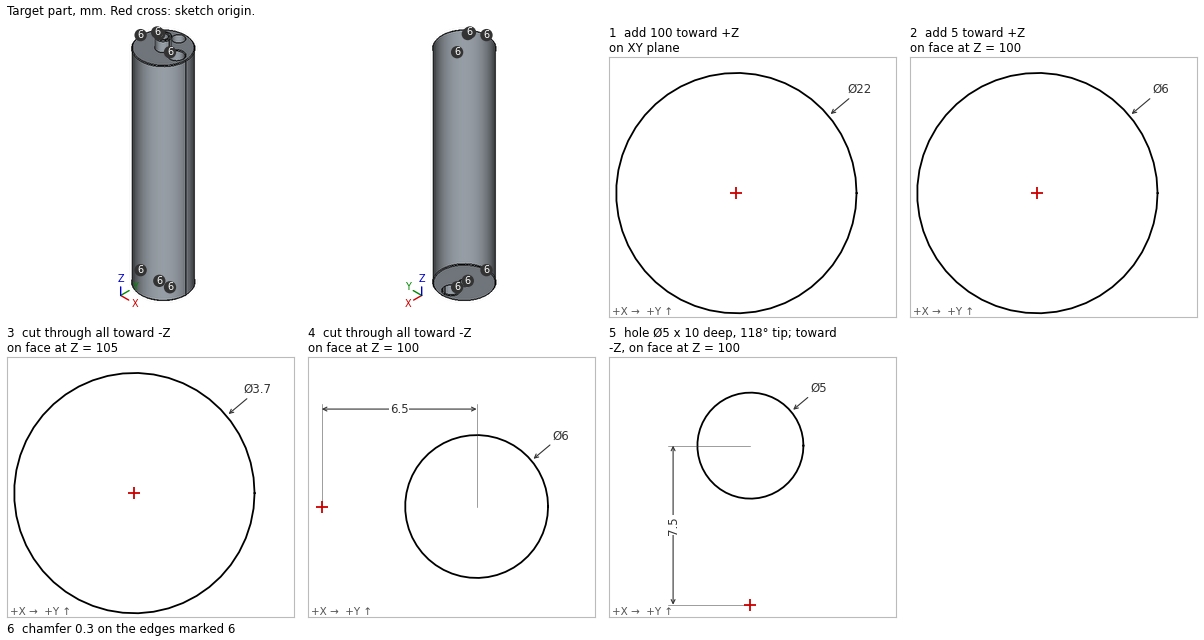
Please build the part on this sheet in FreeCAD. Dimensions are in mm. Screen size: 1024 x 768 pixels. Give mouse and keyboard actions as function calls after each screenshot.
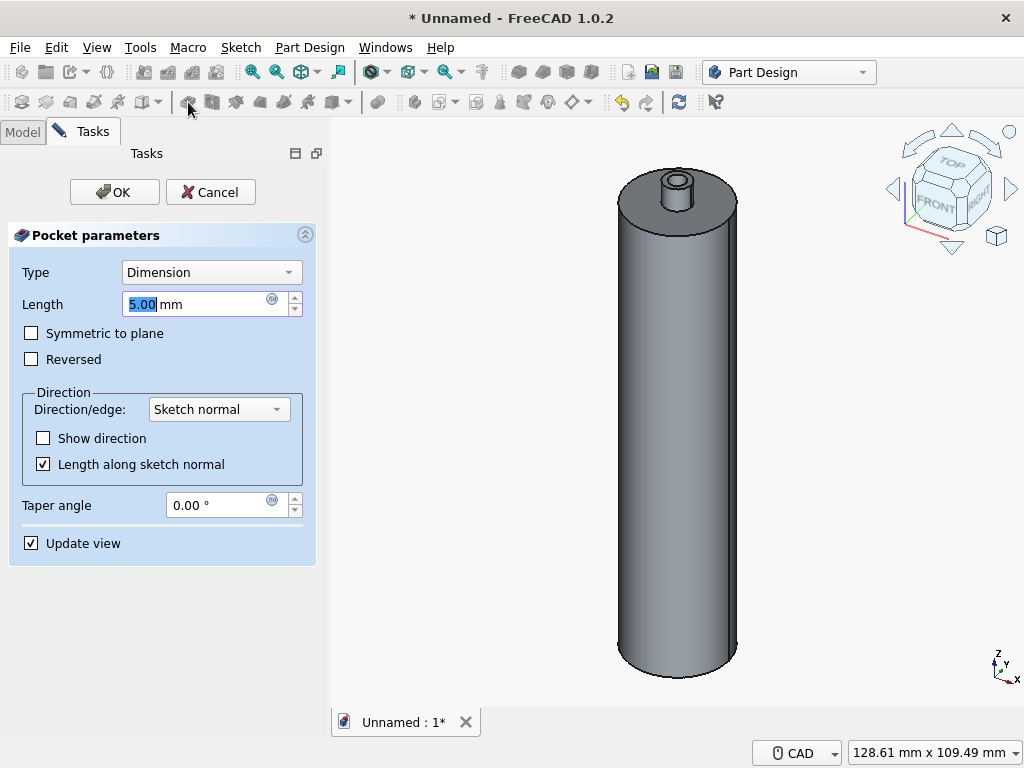
click(212, 272)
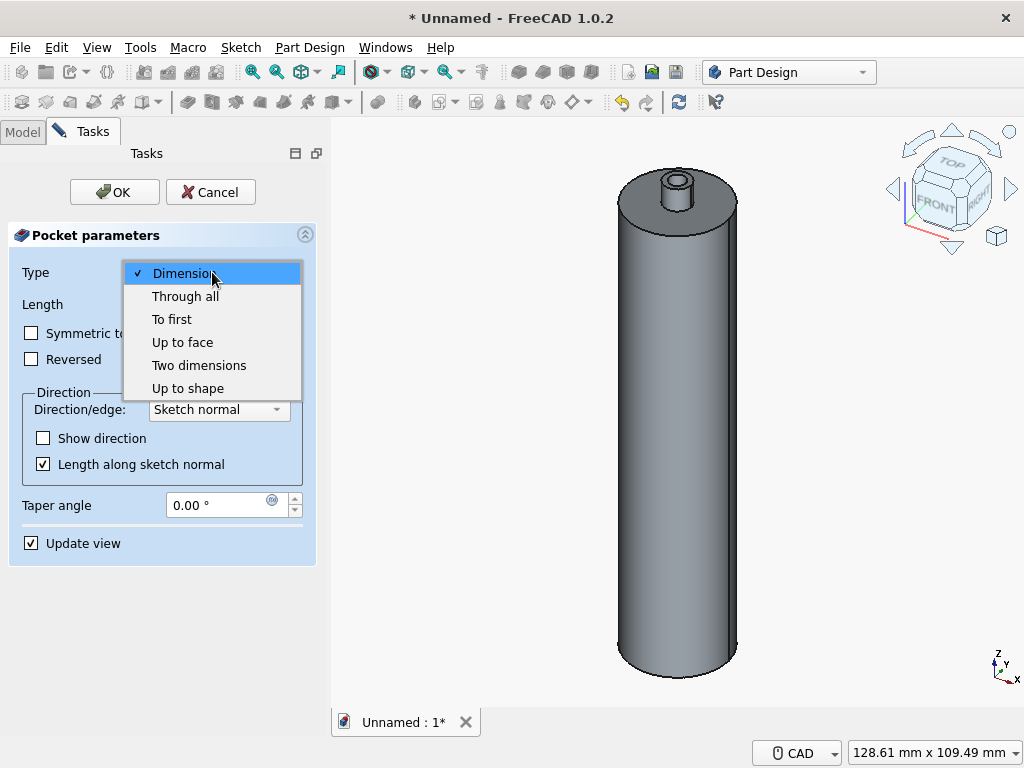
click(212, 296)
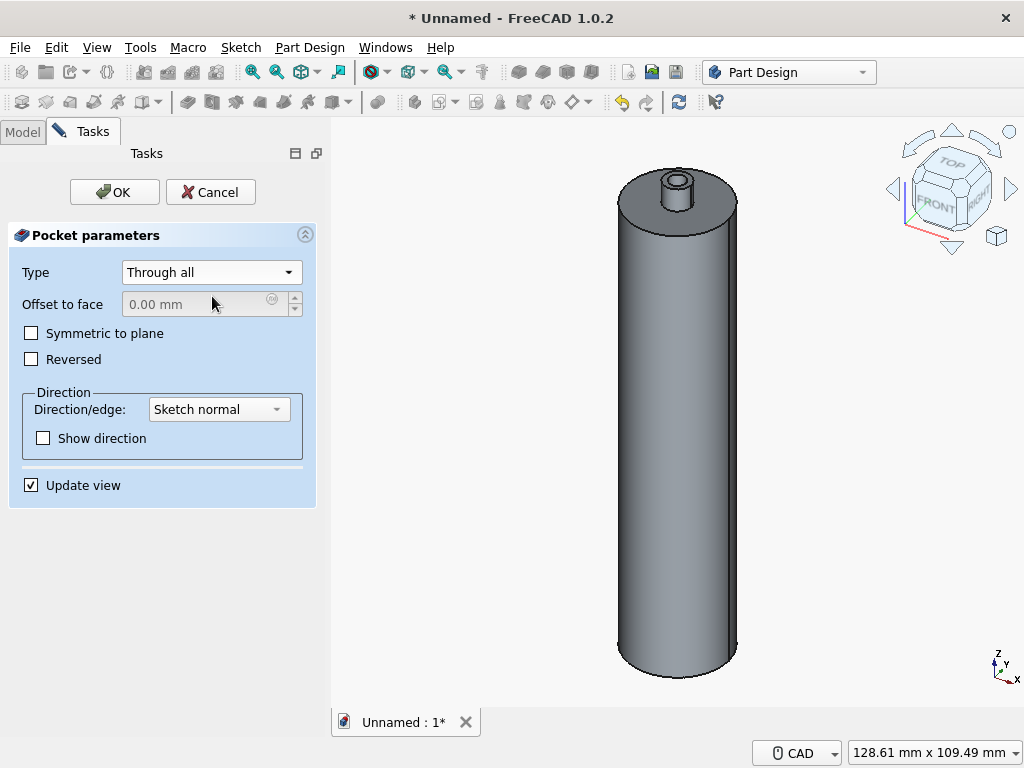
click(115, 192)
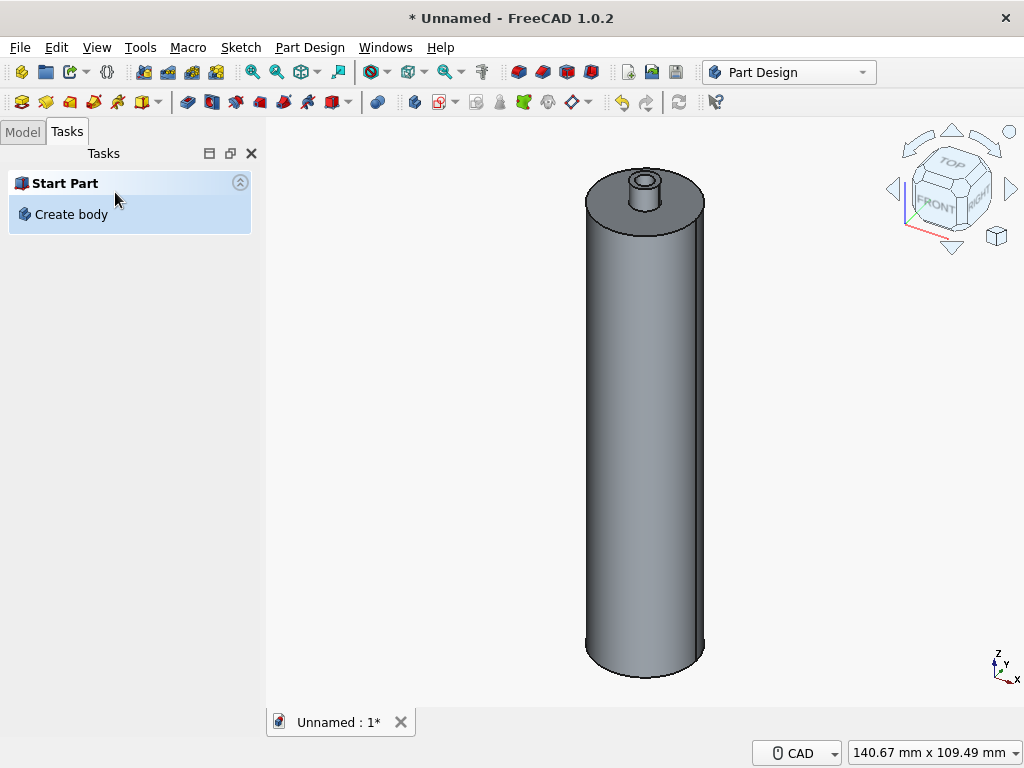
click(677, 189)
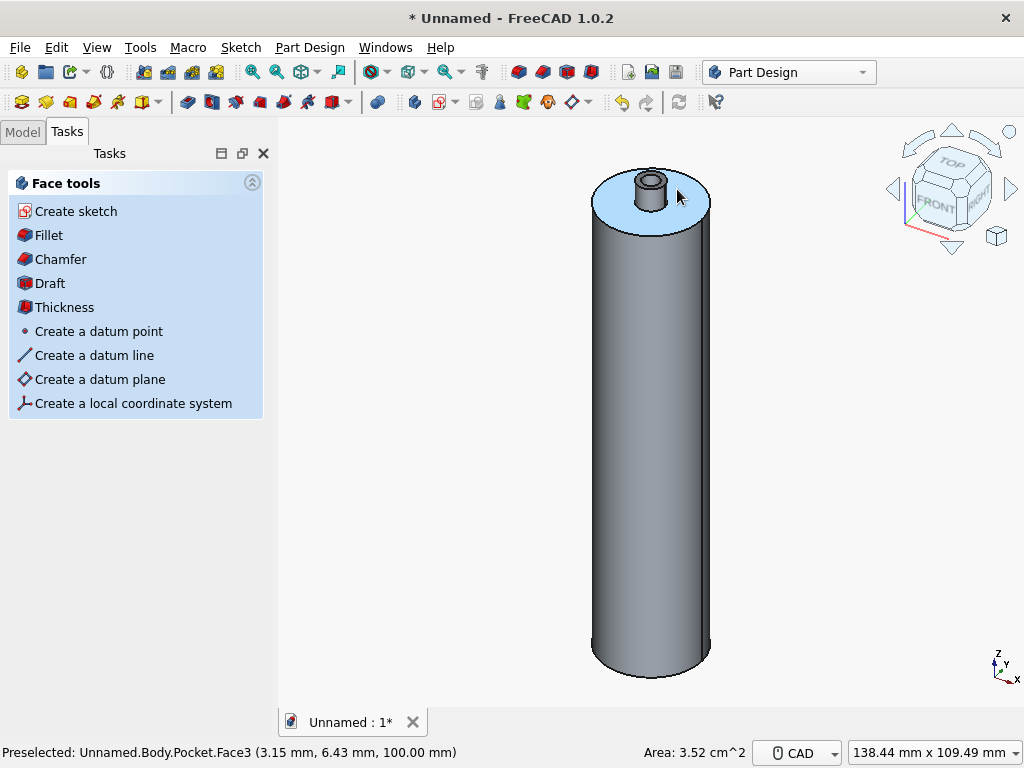
click(440, 102)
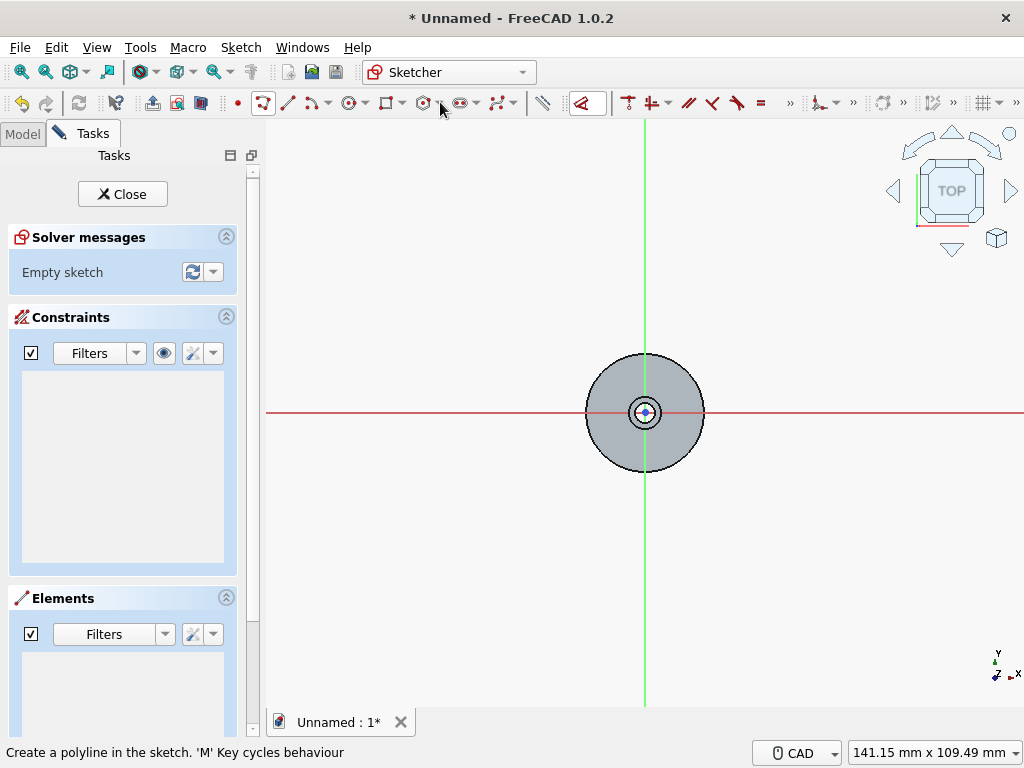
click(202, 104)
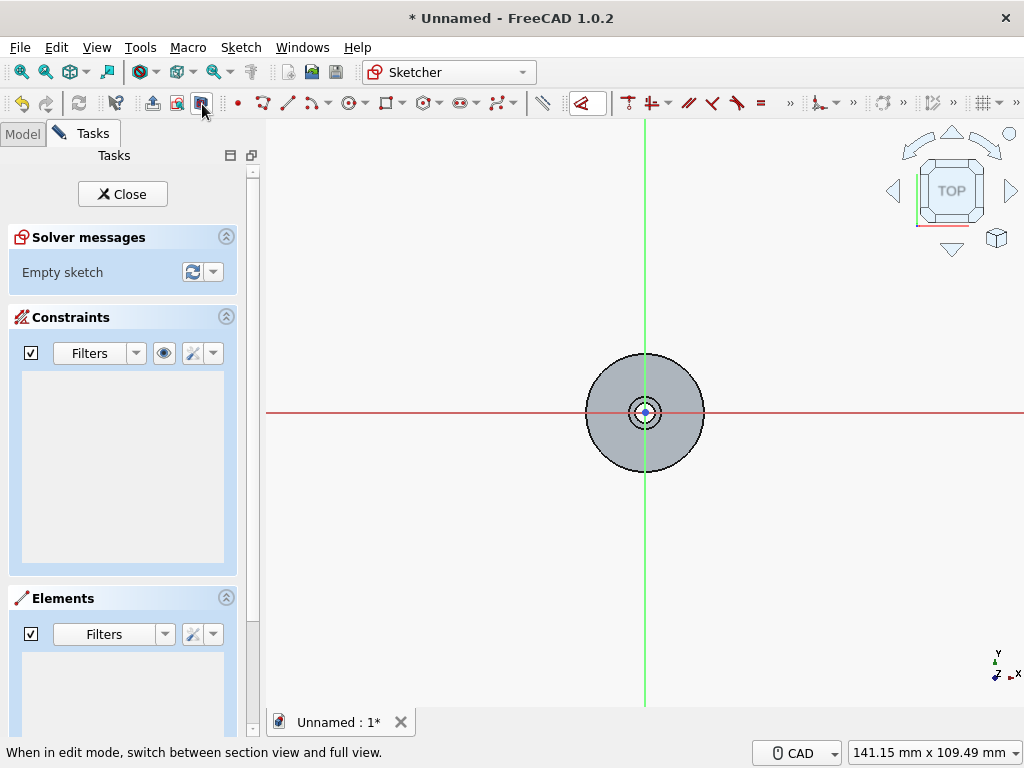
scroll(685, 413, up, 10)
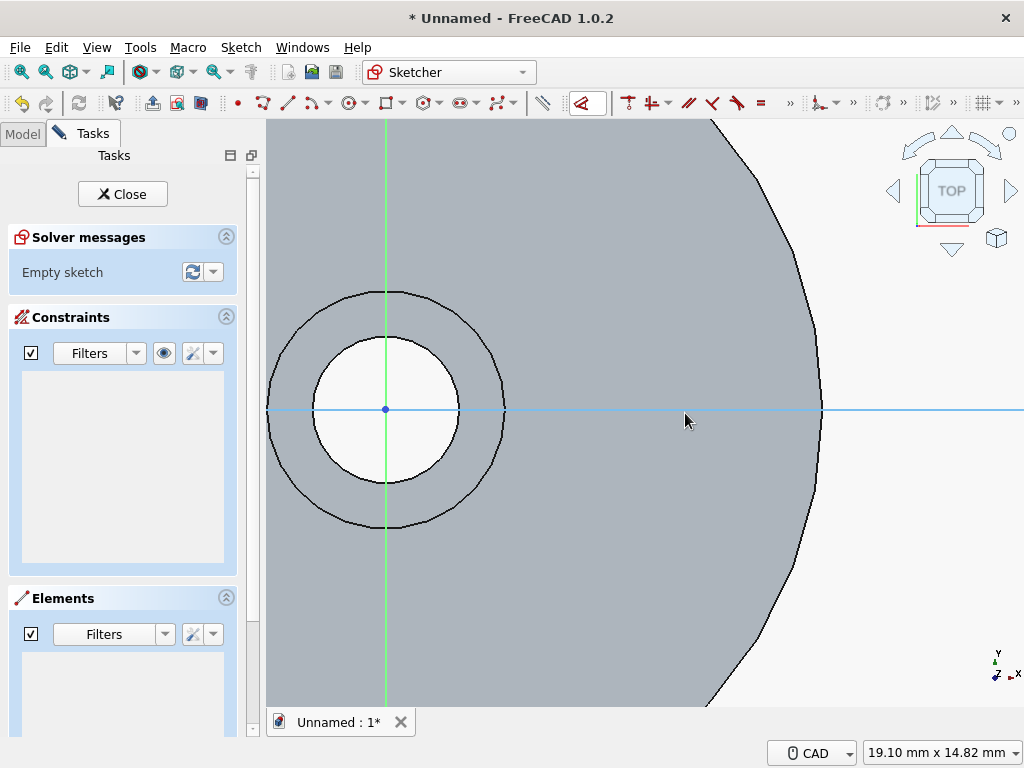
key(g)
key(c)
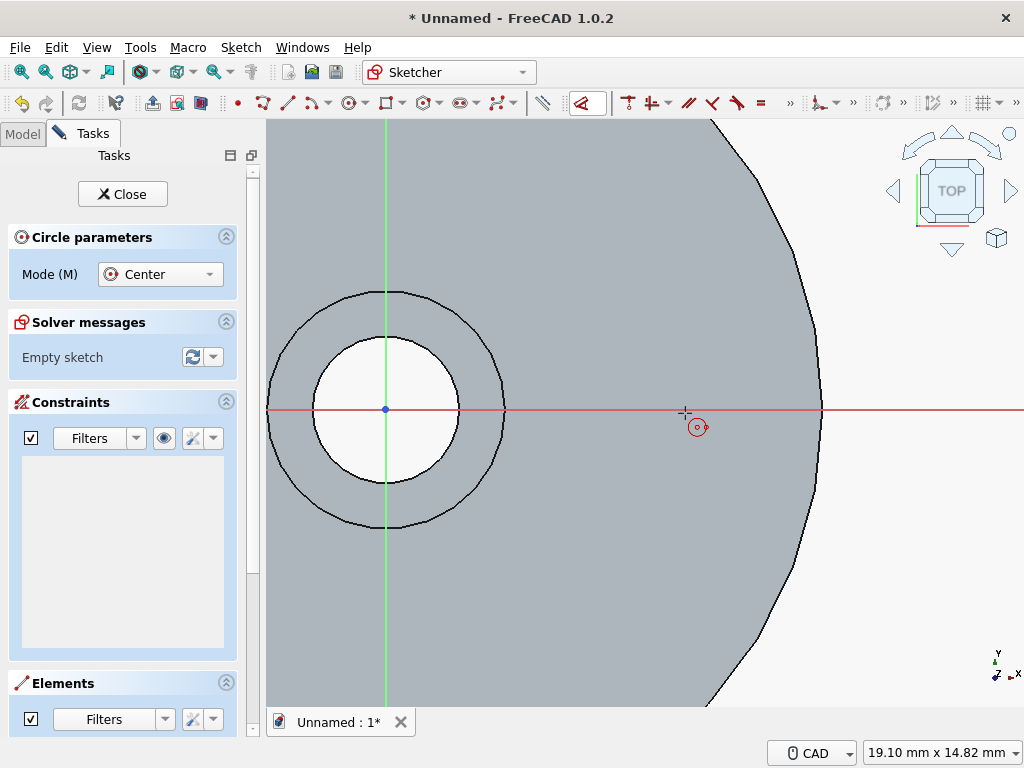
click(644, 410)
click(728, 326)
key(Escape)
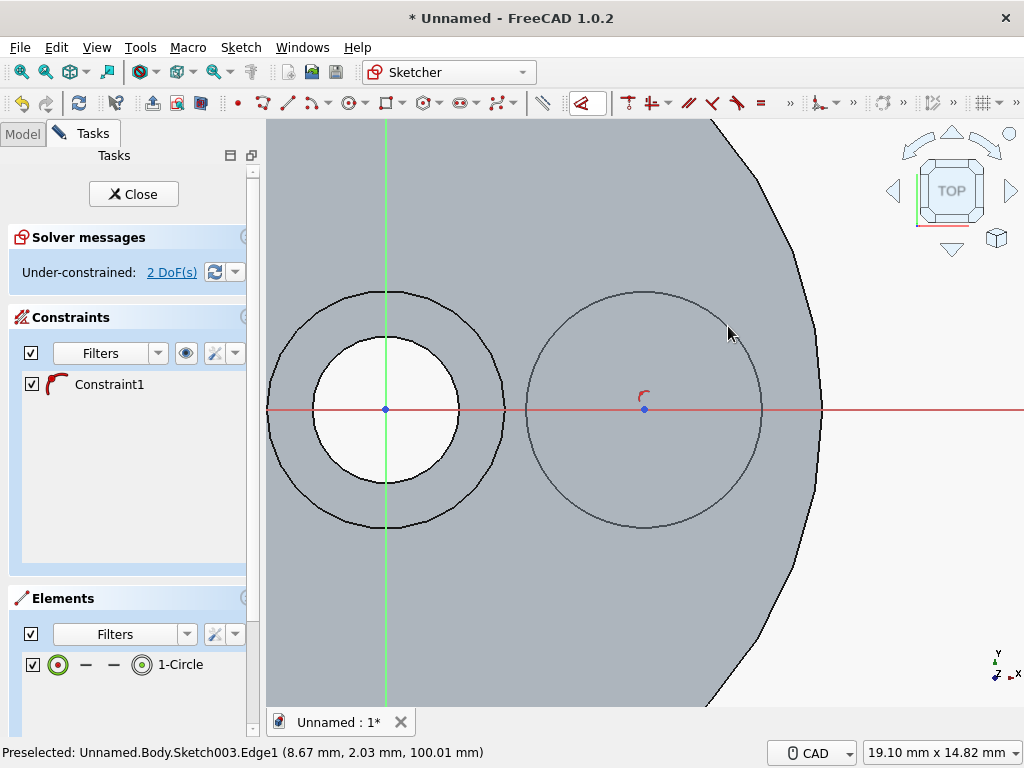
click(727, 326)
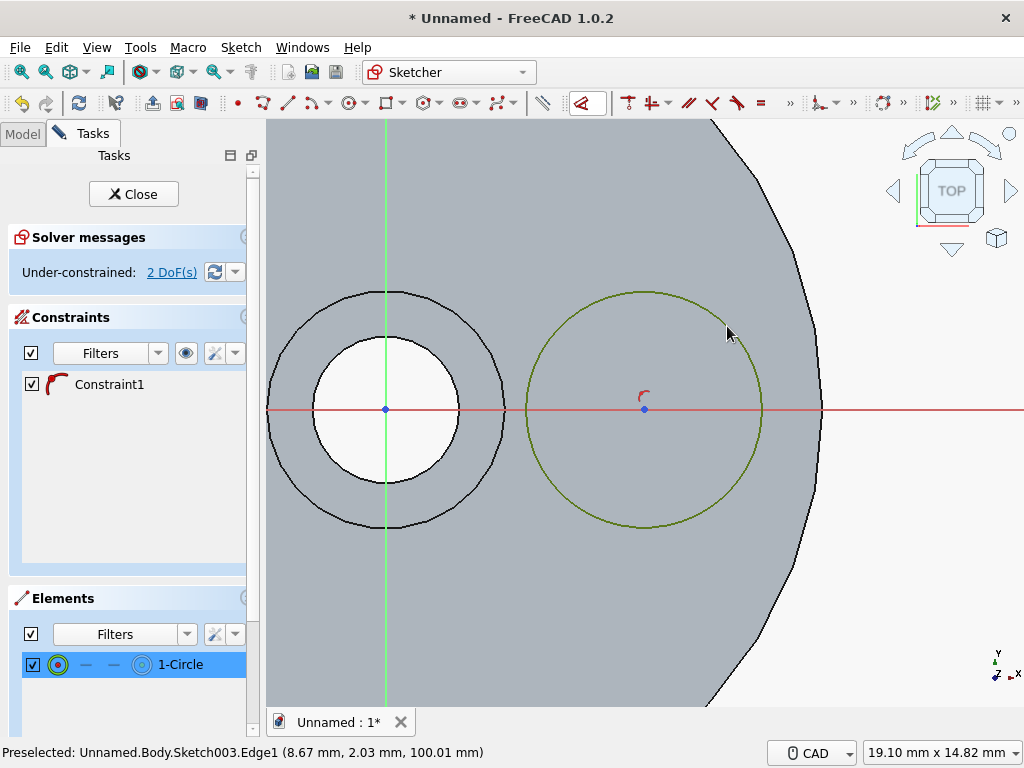
click(600, 104)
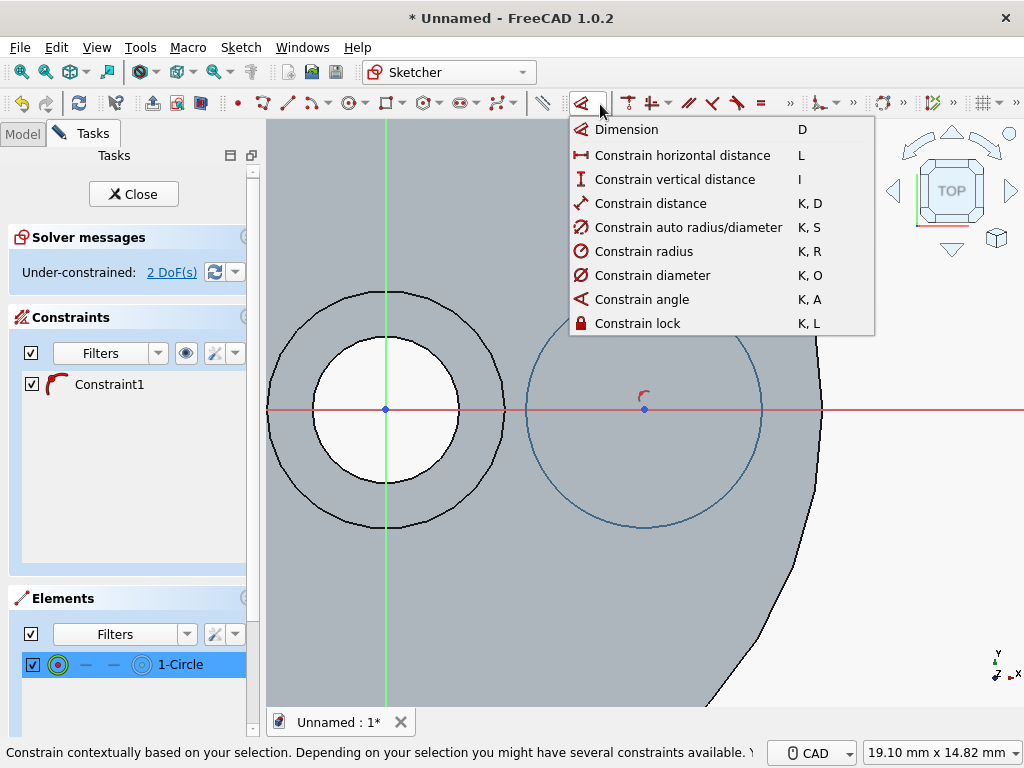
click(722, 275)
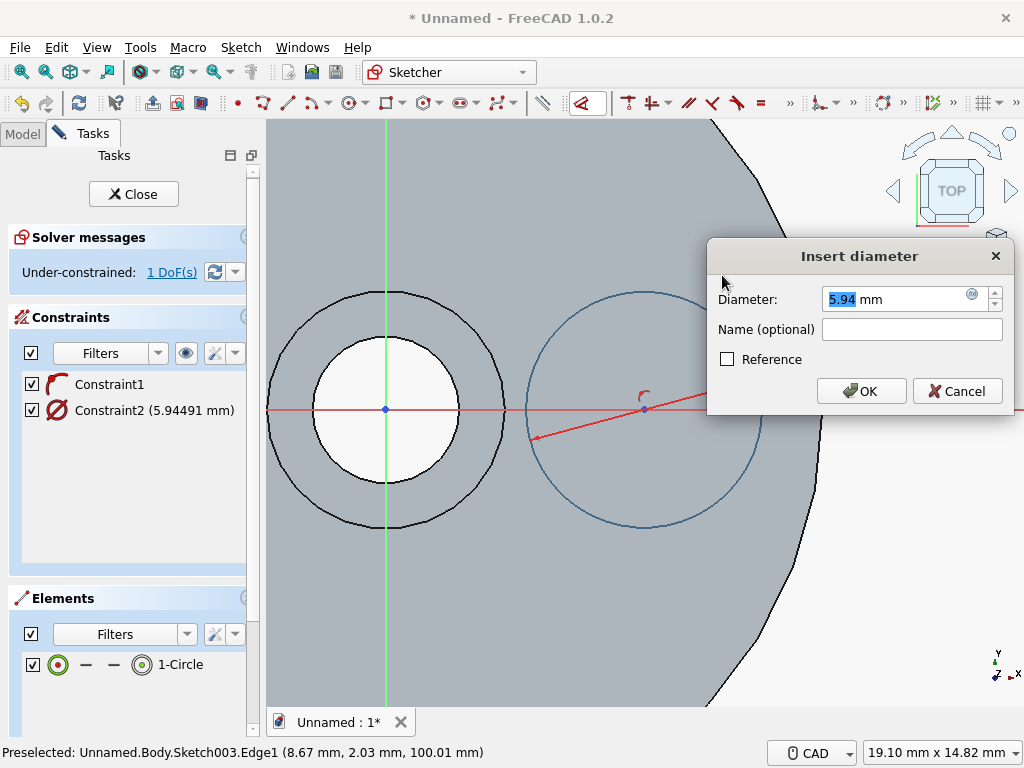
text(6)
key(Return)